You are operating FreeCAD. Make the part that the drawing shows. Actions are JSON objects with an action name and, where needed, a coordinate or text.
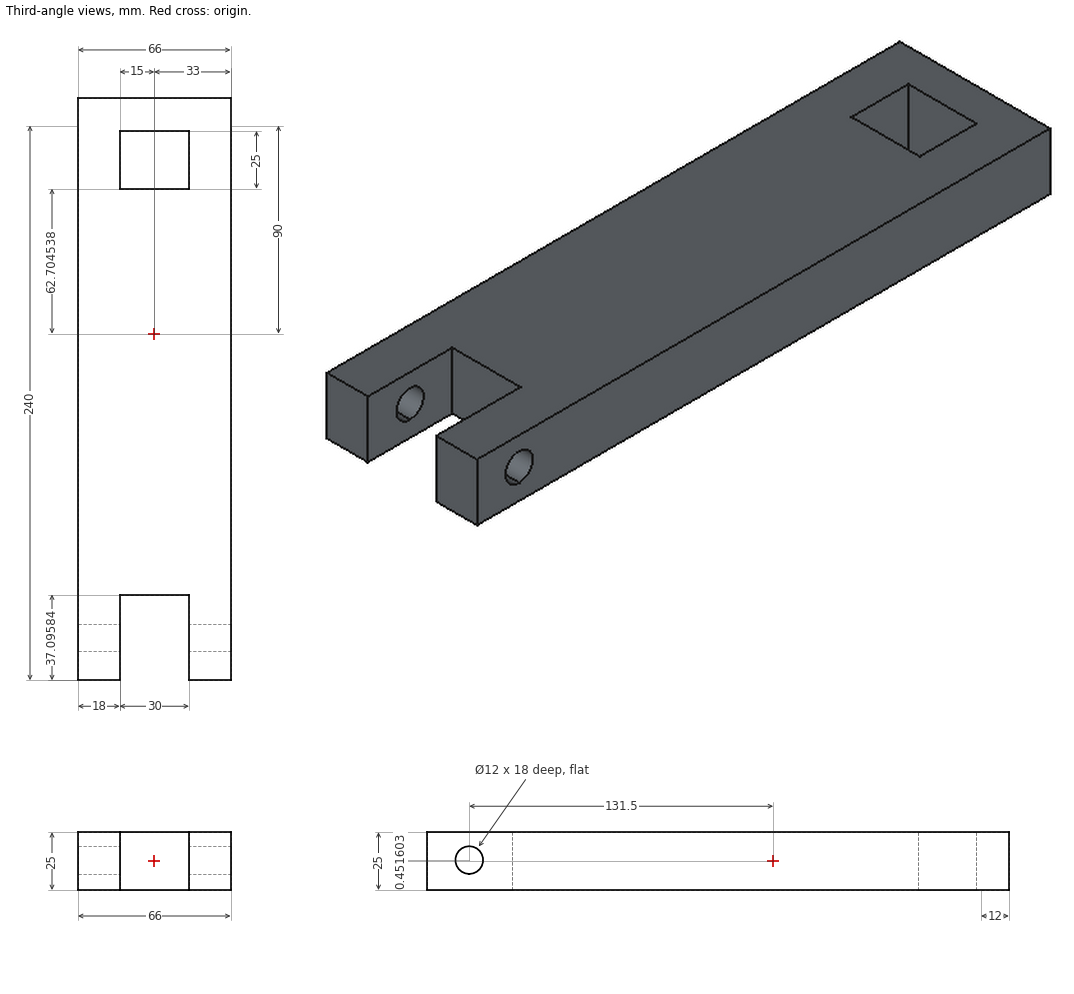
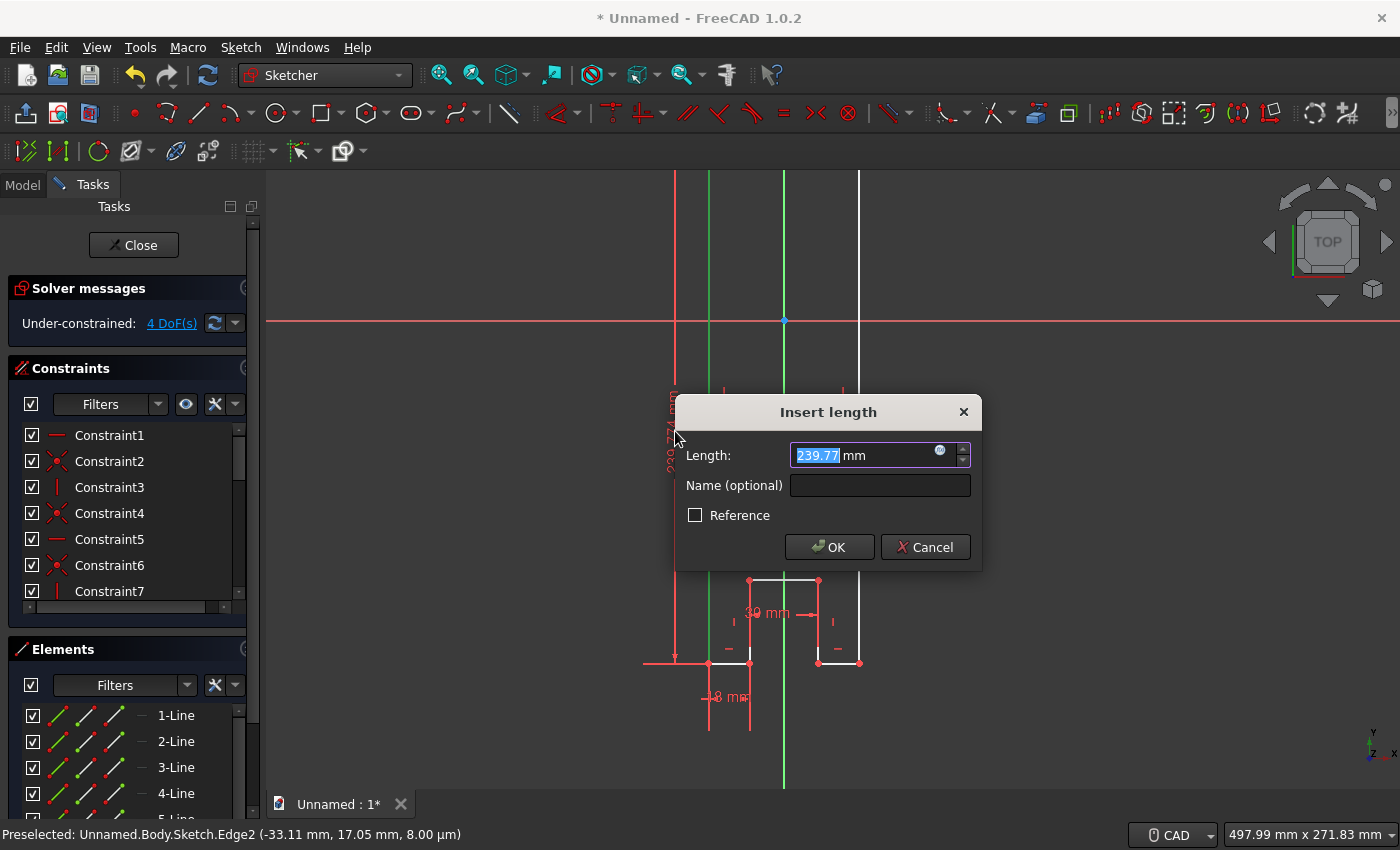
{"action": "type", "text": "240"}
{"action": "key", "text": "Return"}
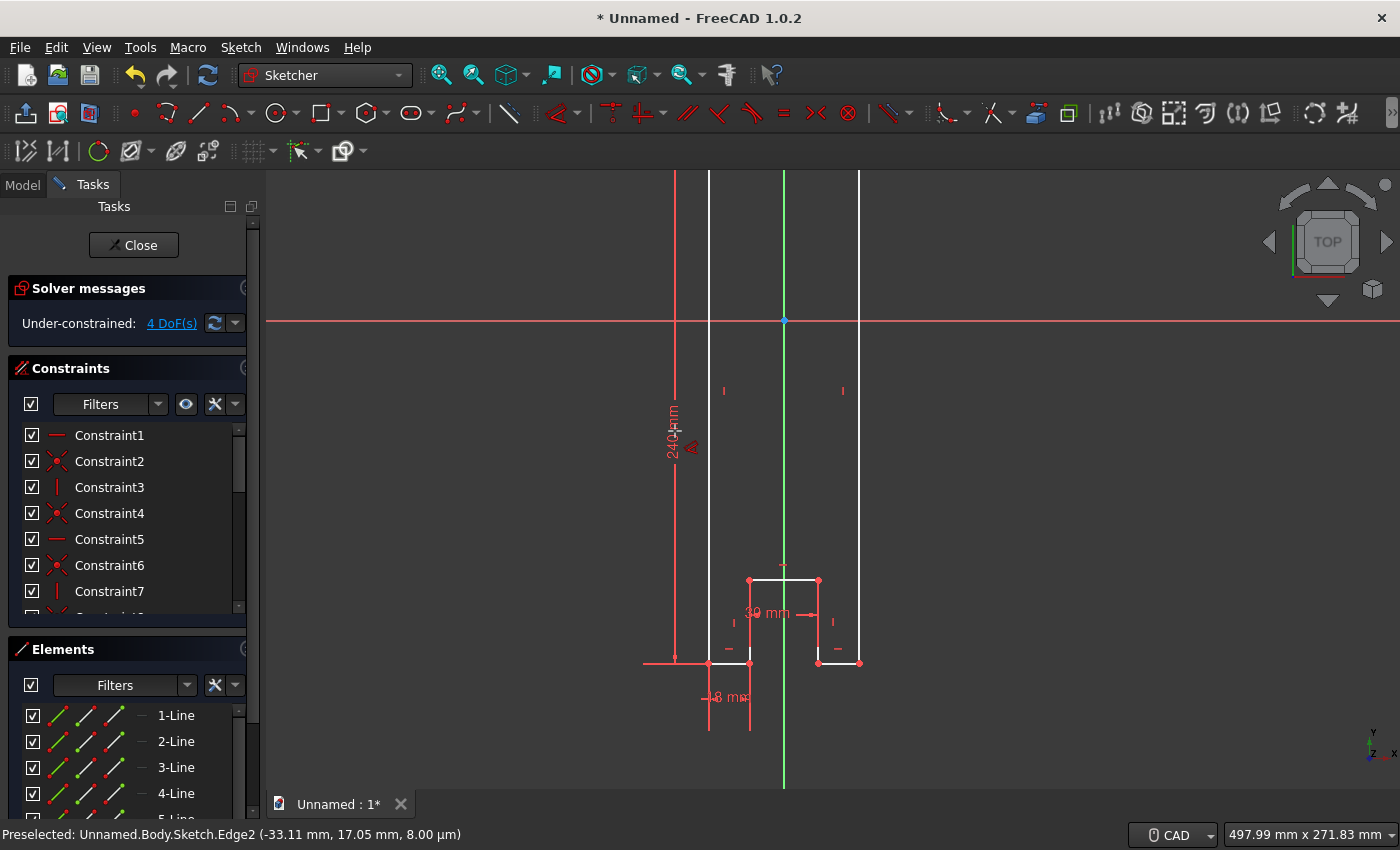
{"action": "left_click", "coordinate": [859, 500]}
{"action": "left_click", "coordinate": [893, 431]}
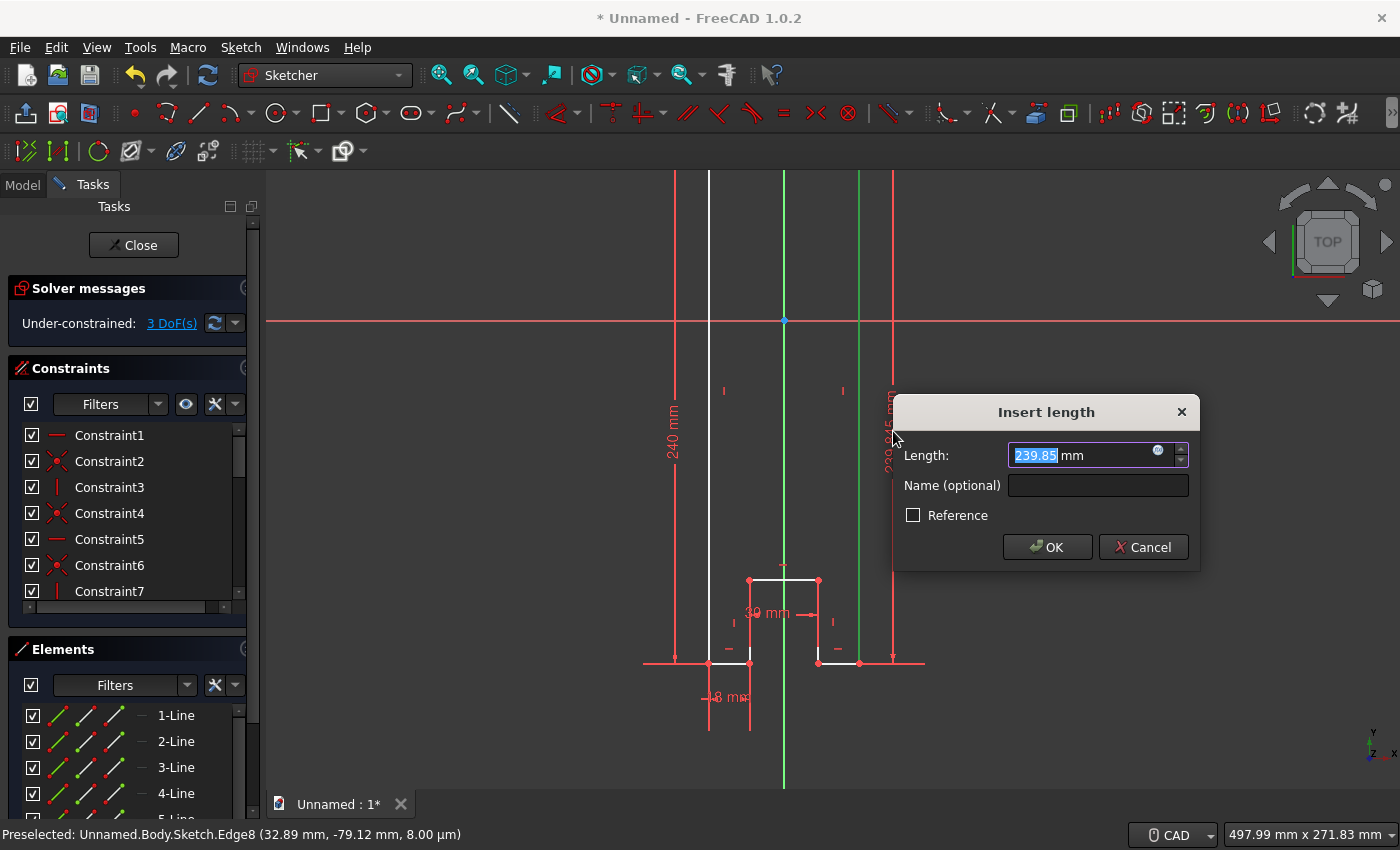
{"action": "type", "text": "240"}
{"action": "key", "text": "Return"}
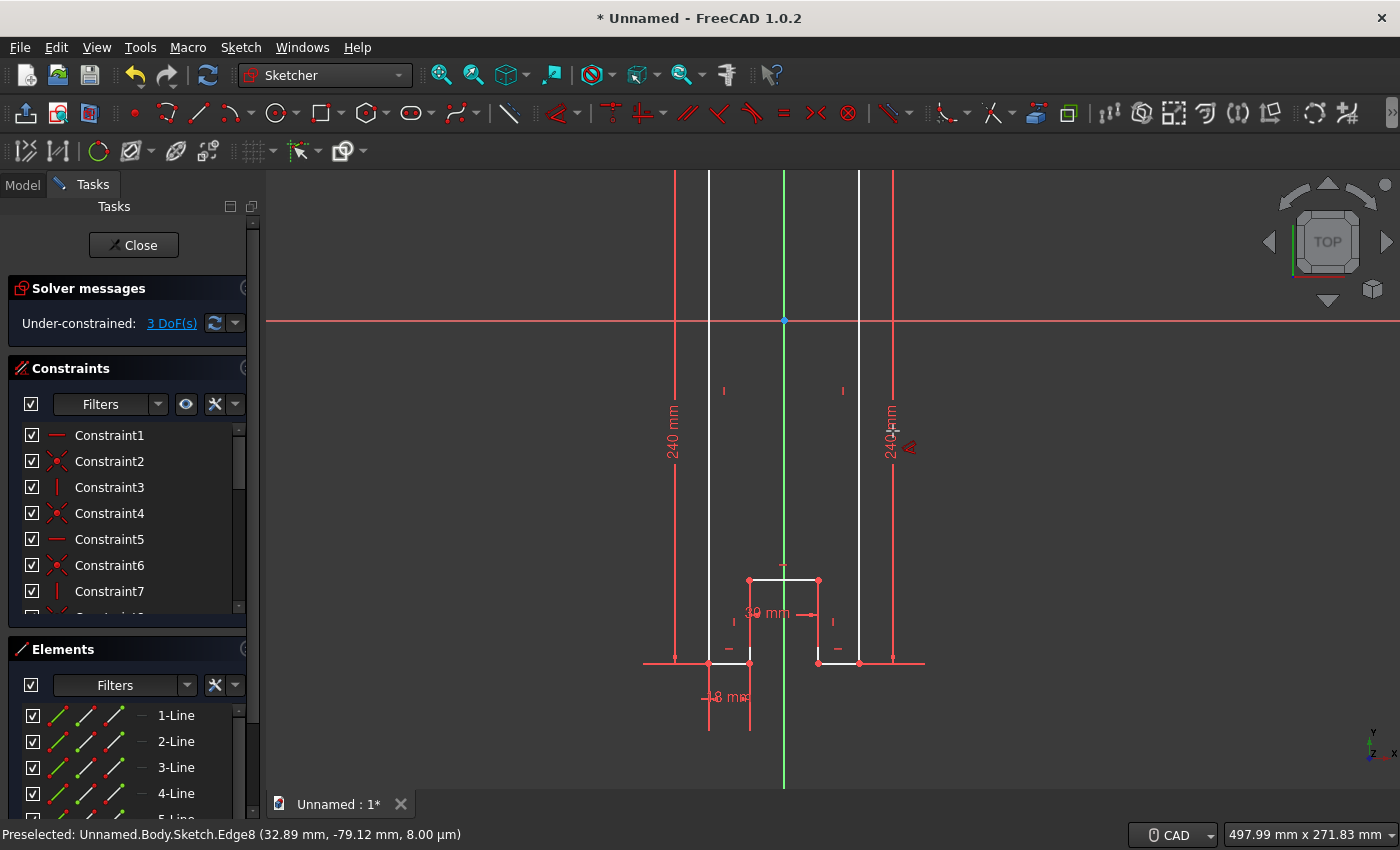
{"action": "scroll", "coordinate": [725, 663], "scroll_direction": "down", "scroll_amount": 2}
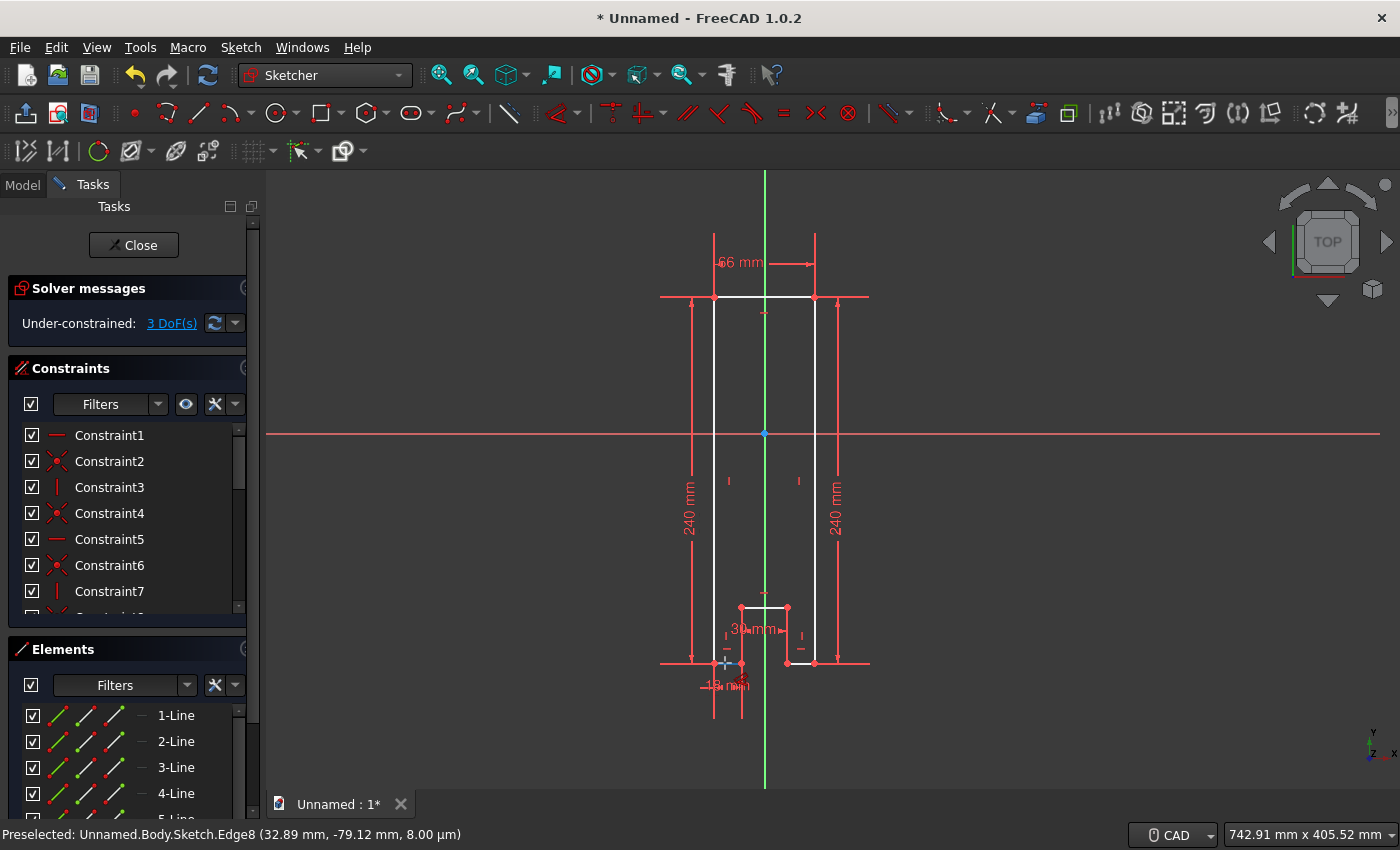
{"action": "left_click", "coordinate": [815, 297]}
{"action": "left_click", "coordinate": [790, 468]}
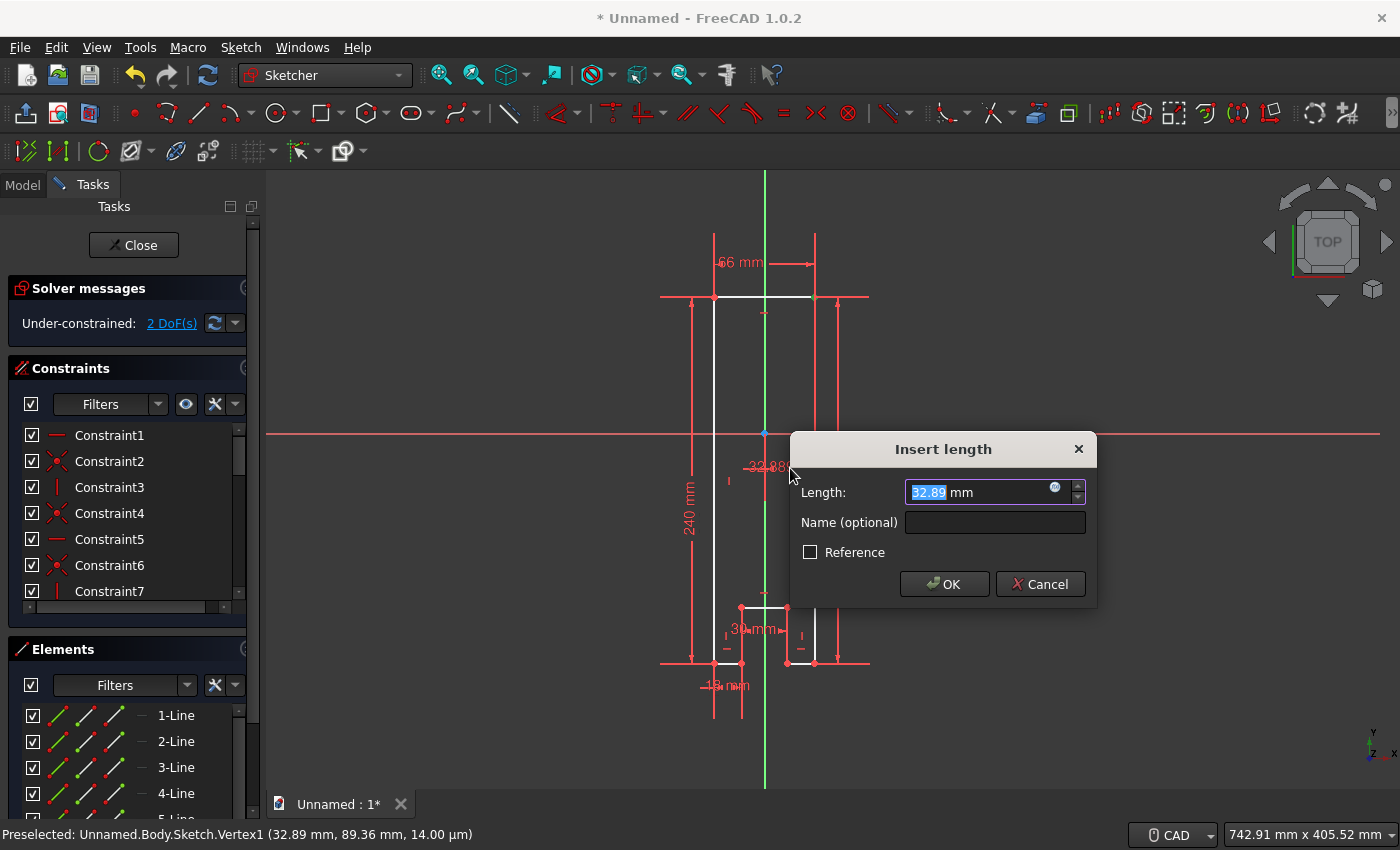
{"action": "type", "text": "33"}
{"action": "key", "text": "Return"}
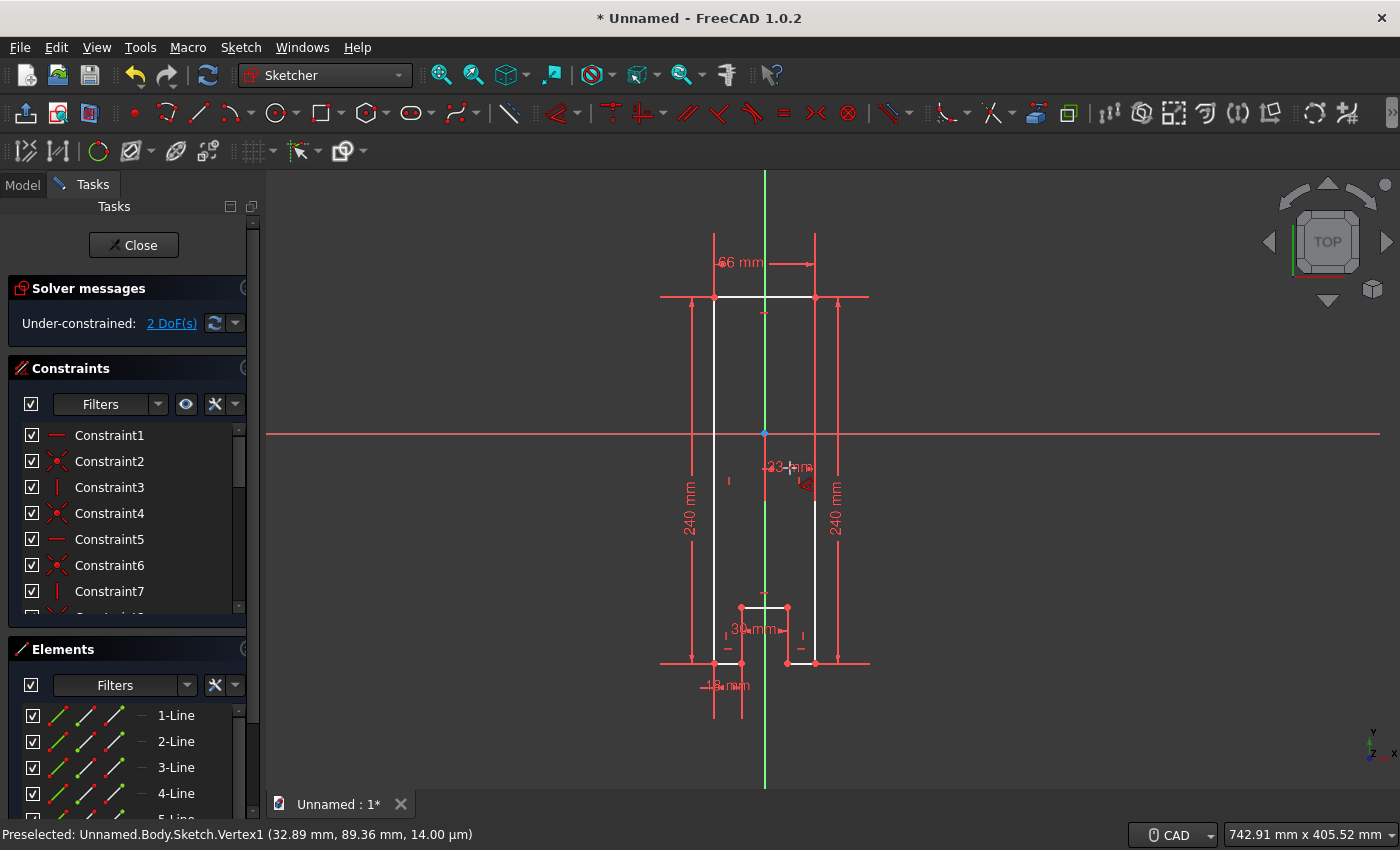
{"action": "left_click", "coordinate": [815, 297]}
{"action": "left_click", "coordinate": [849, 366]}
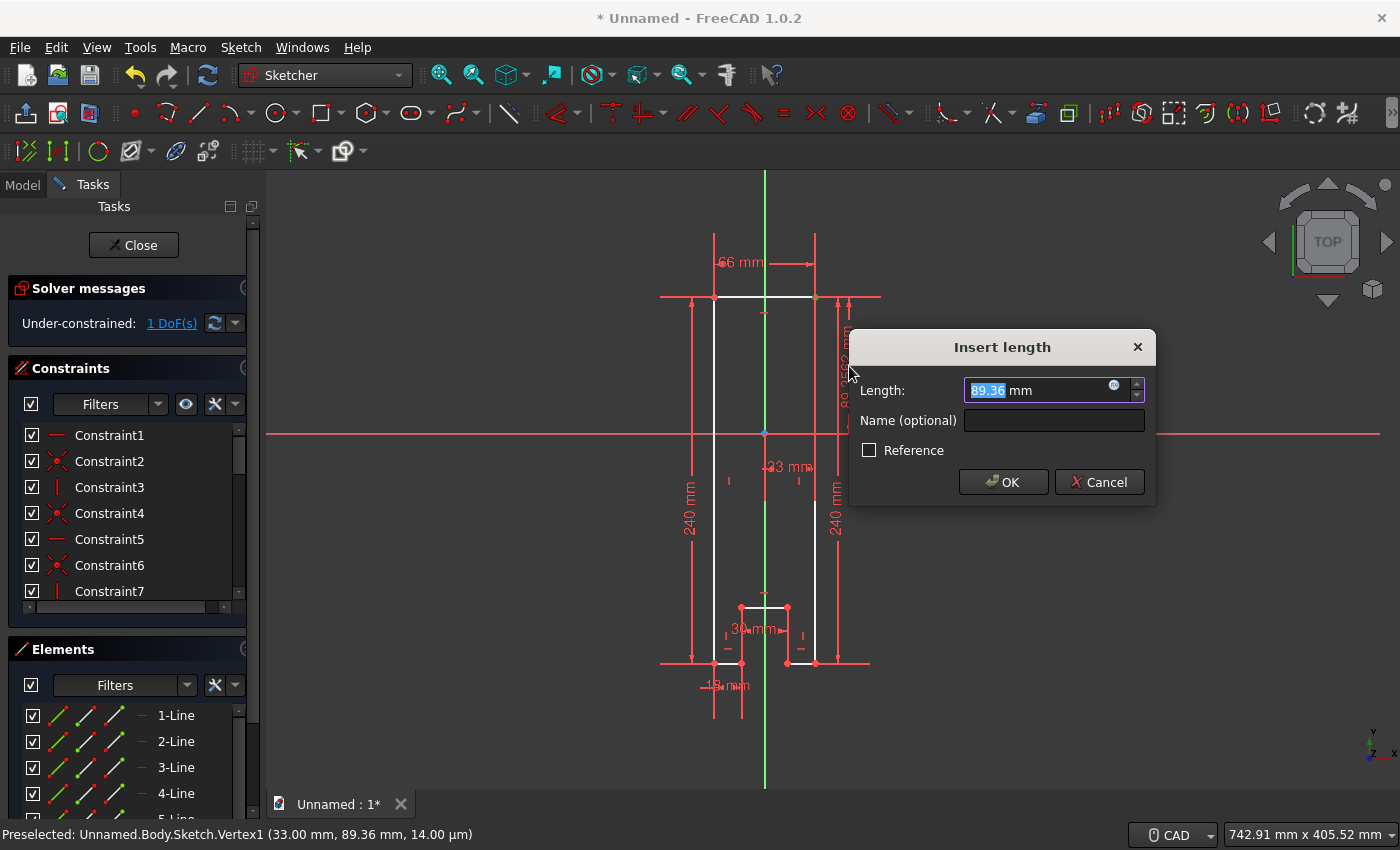
{"action": "type", "text": "90"}
{"action": "key", "text": "Return"}